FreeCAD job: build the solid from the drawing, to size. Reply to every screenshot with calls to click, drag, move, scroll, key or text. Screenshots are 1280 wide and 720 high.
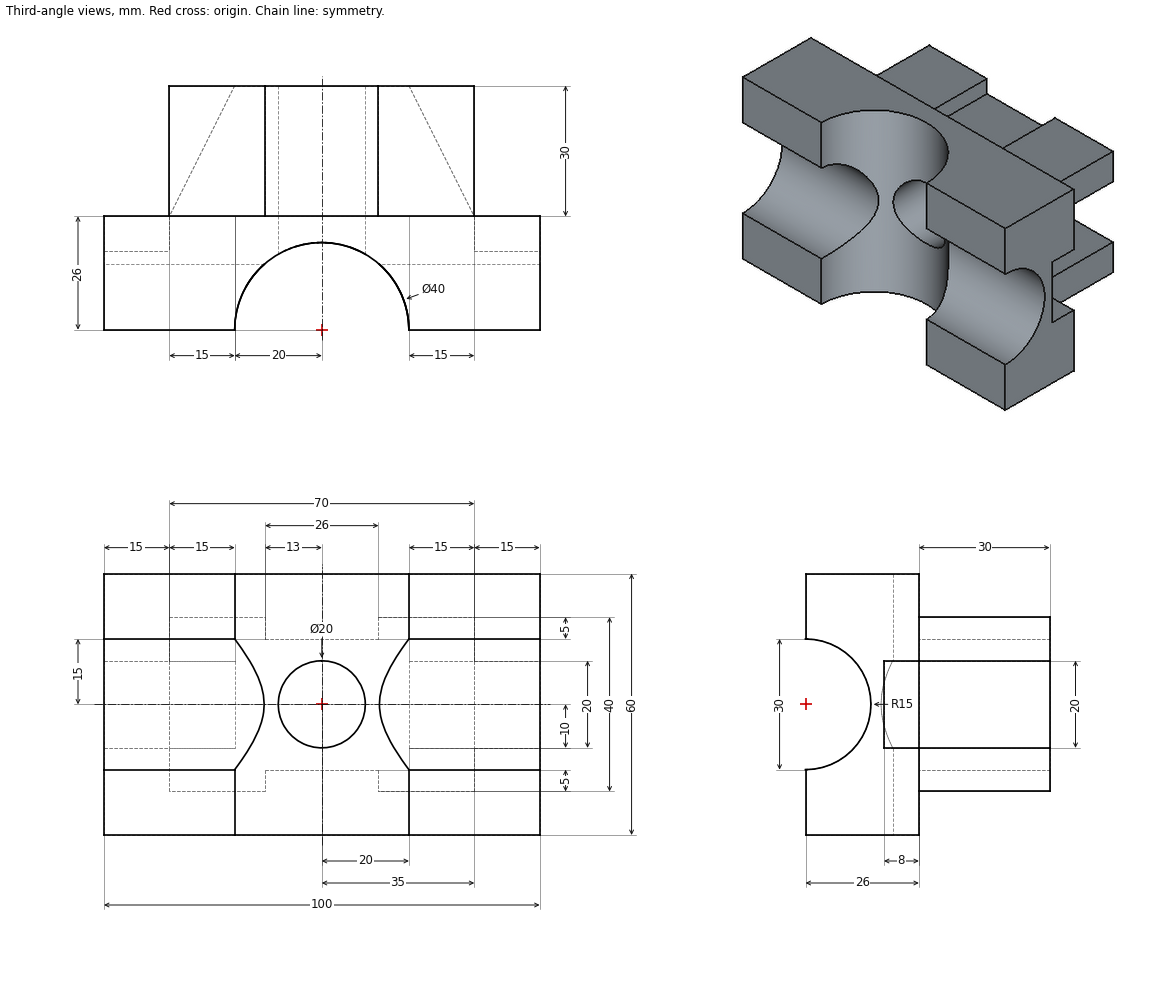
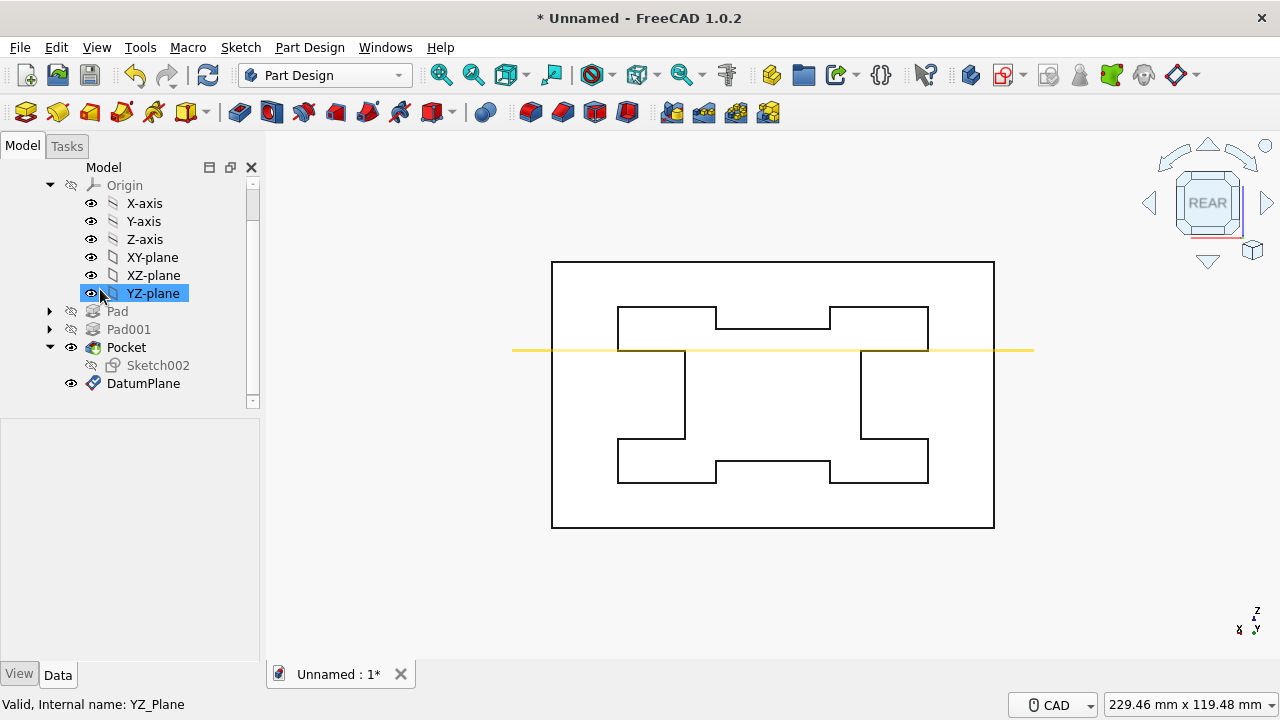
click(116, 383)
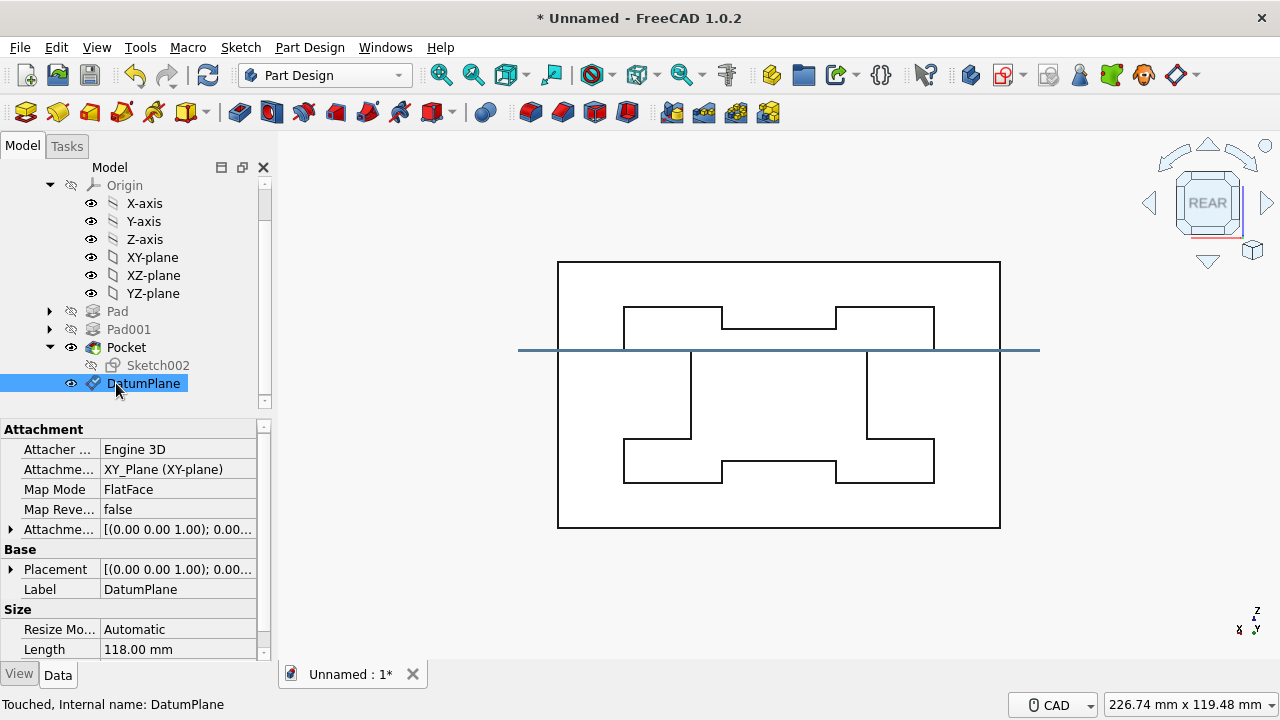
click(1004, 76)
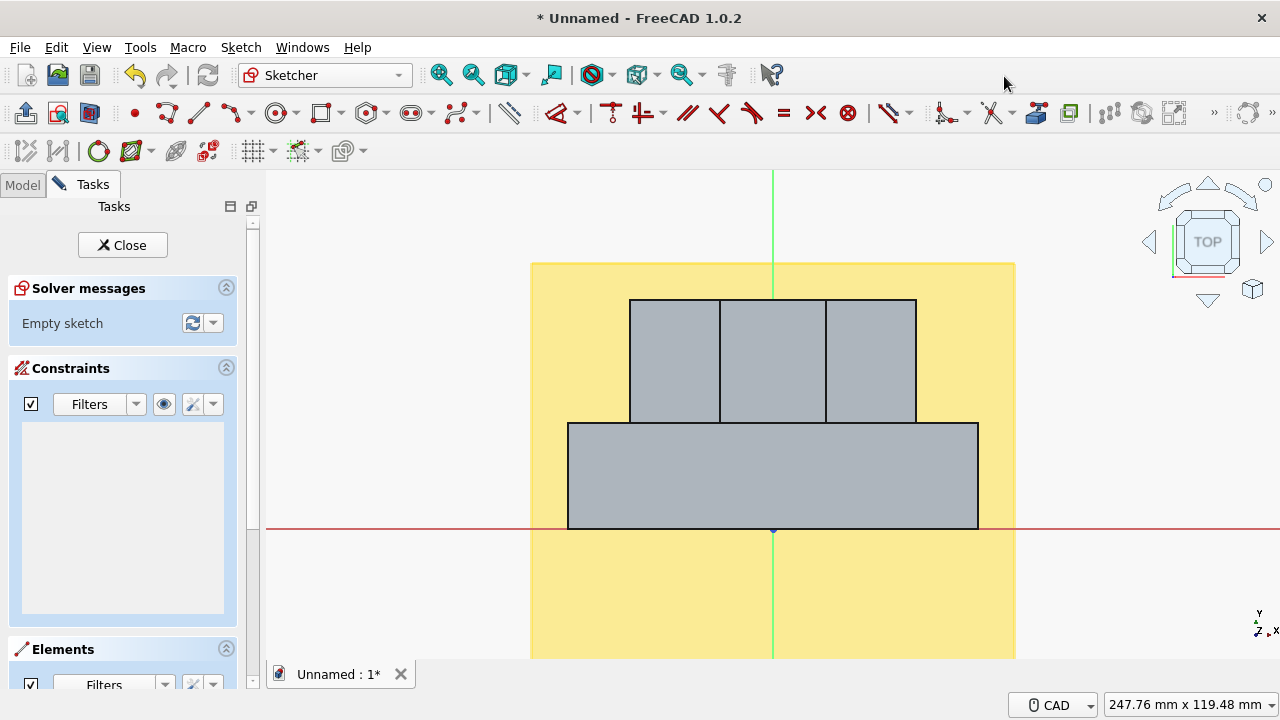
click(90, 114)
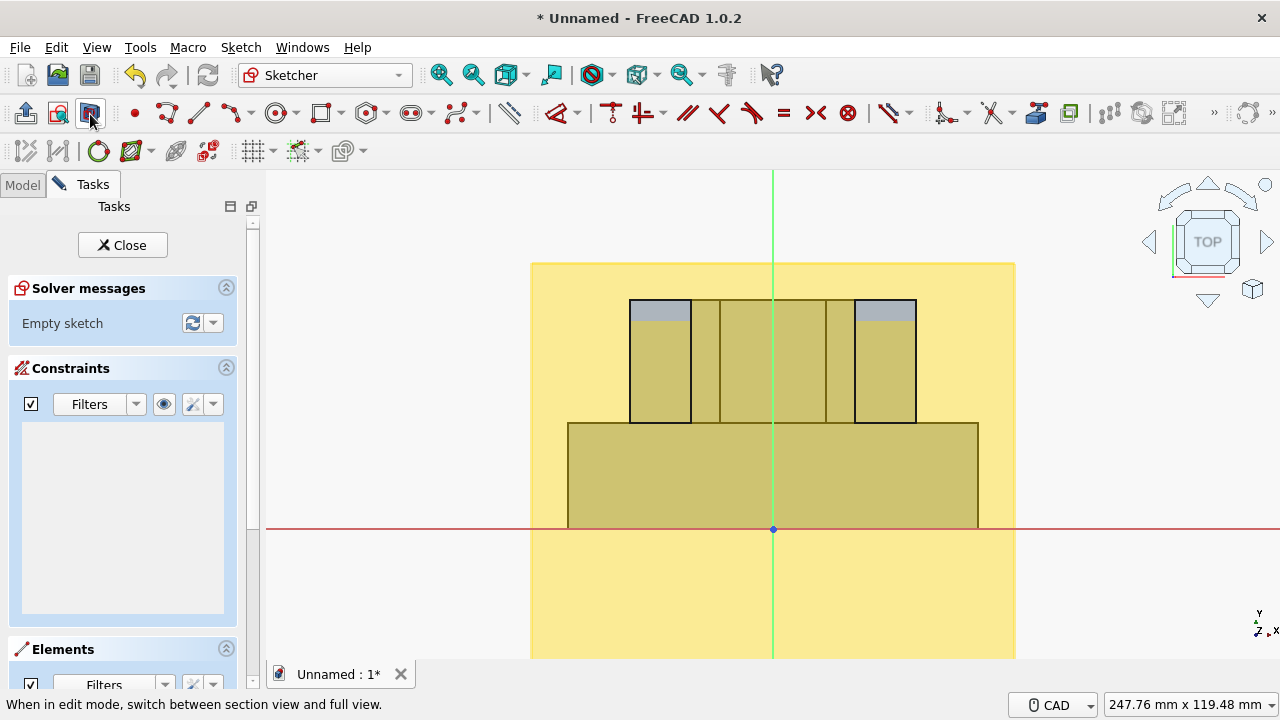
key(g)
key(m)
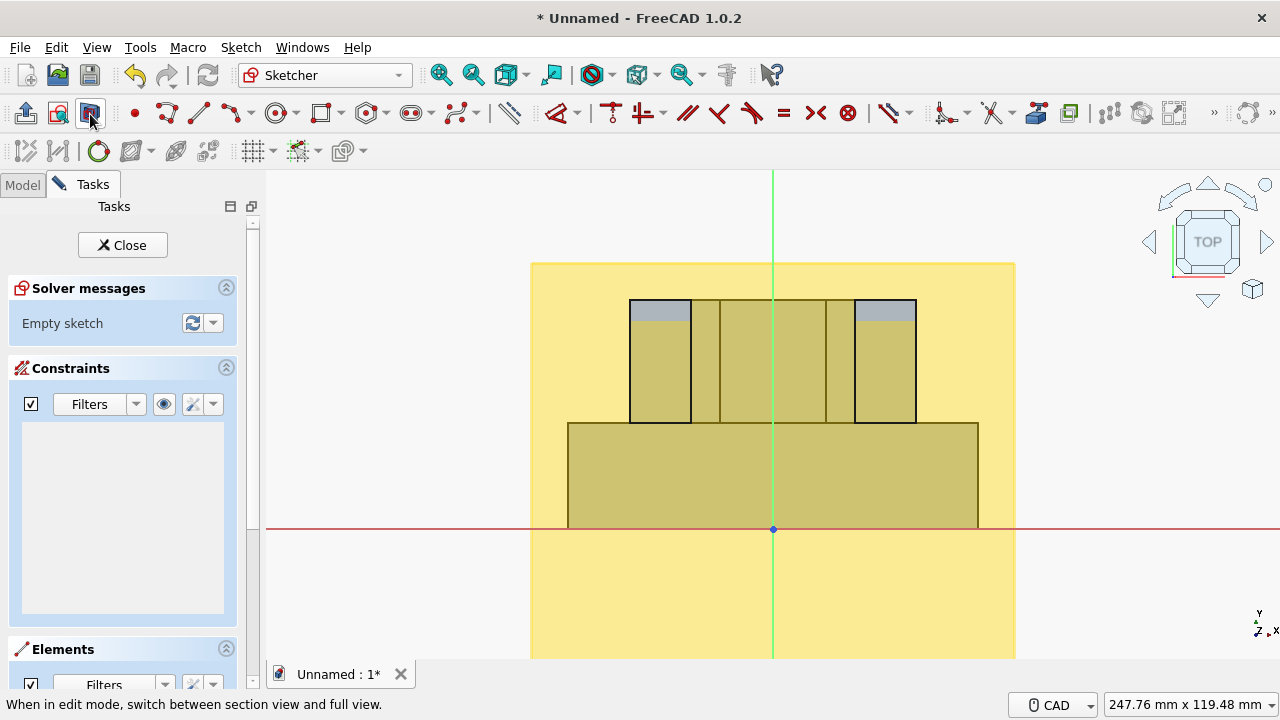
click(691, 423)
click(691, 300)
click(630, 423)
click(691, 424)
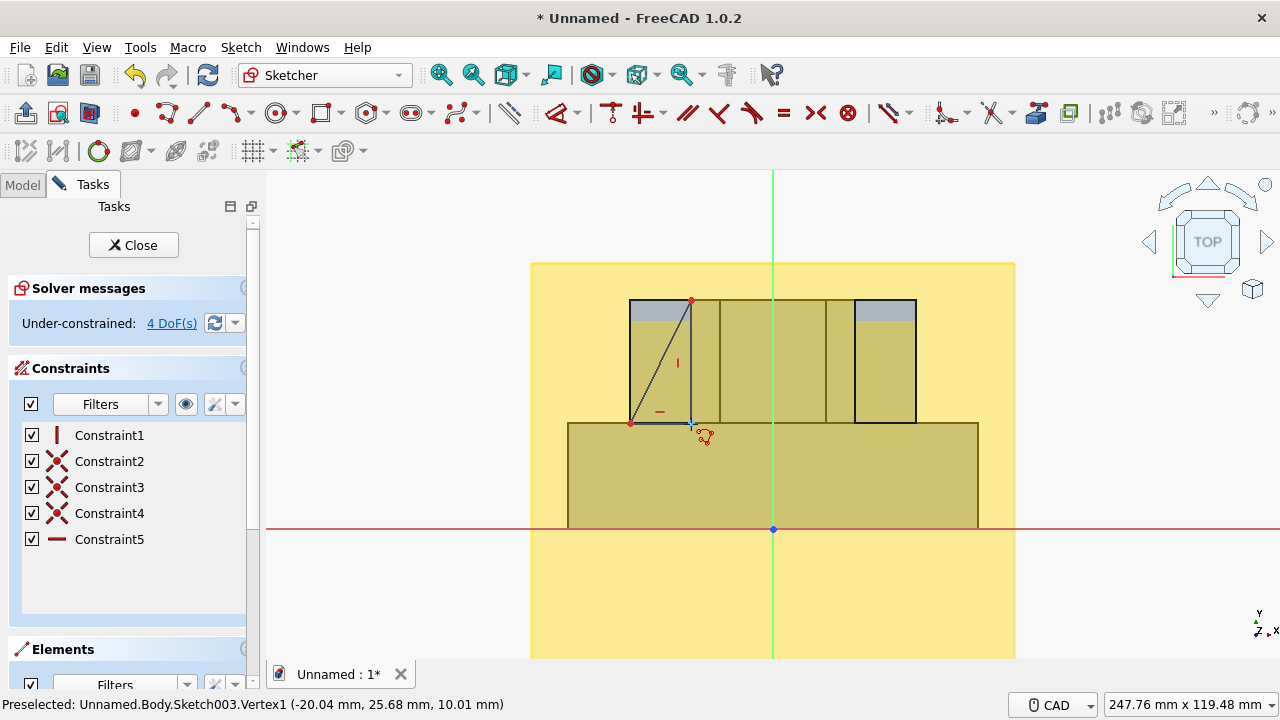
click(855, 423)
click(916, 423)
click(855, 300)
click(855, 424)
key(Escape)
key(Escape)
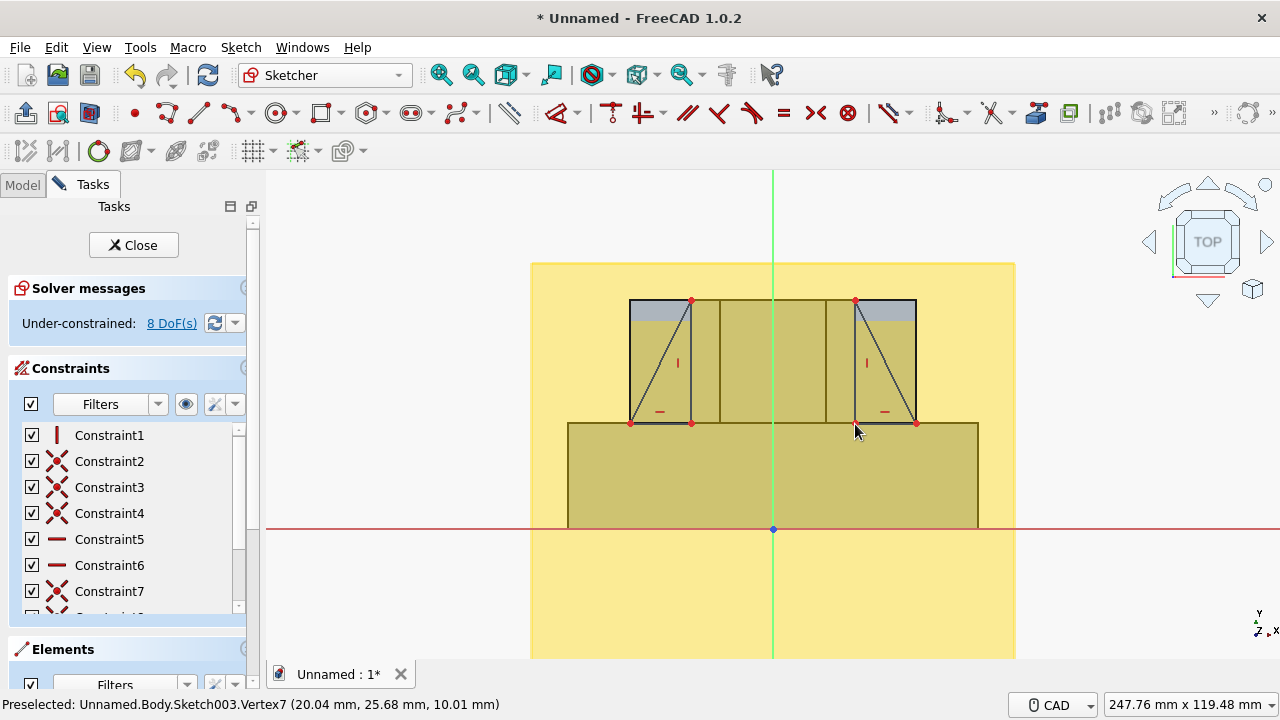
click(691, 424)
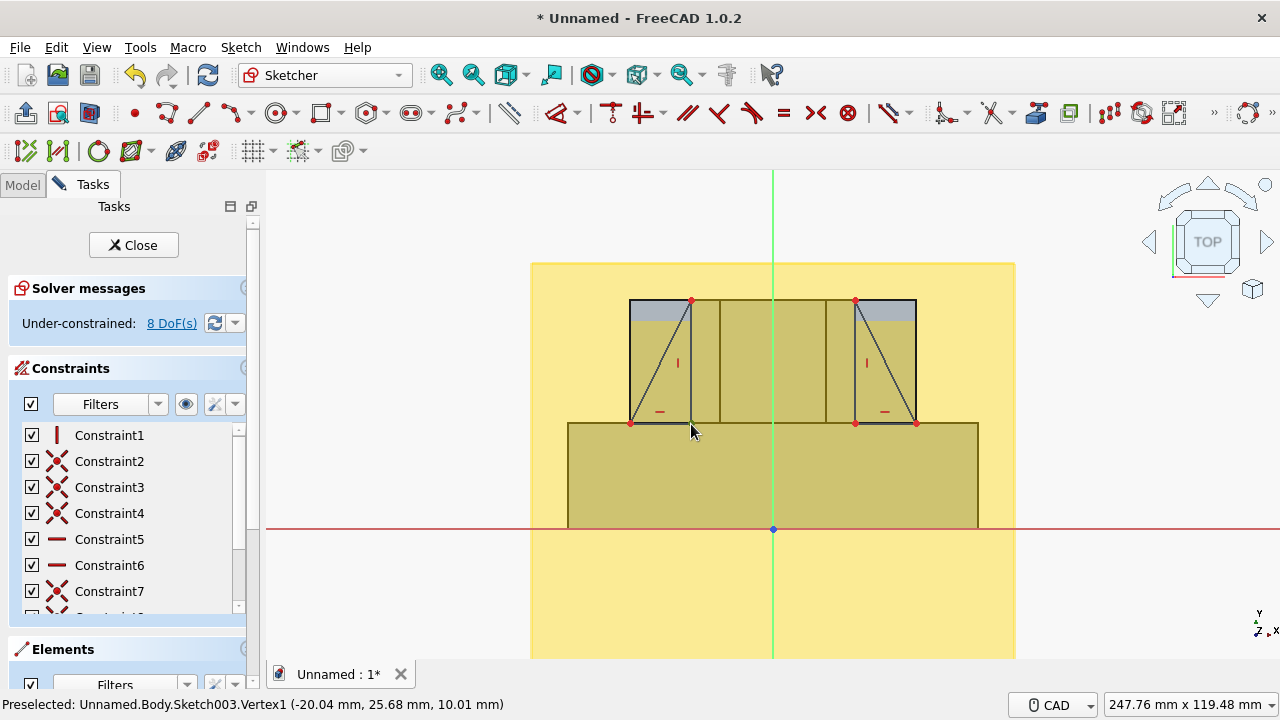
click(855, 424)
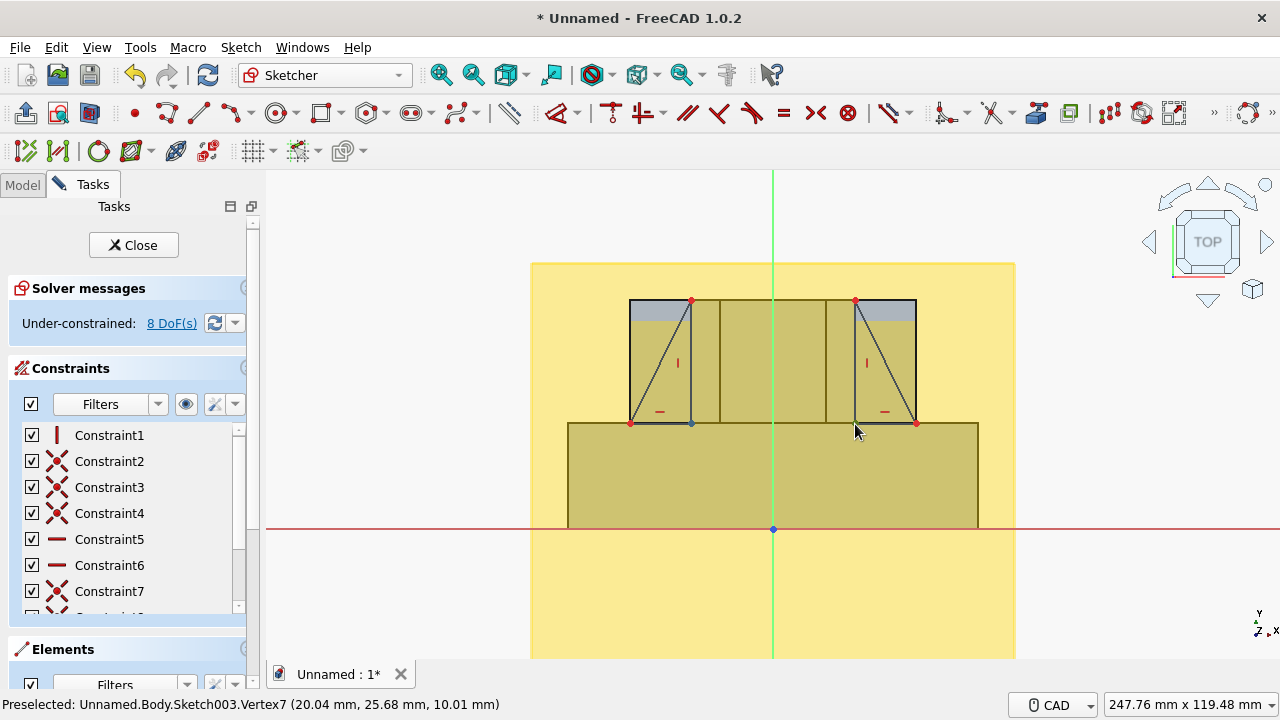
click(773, 600)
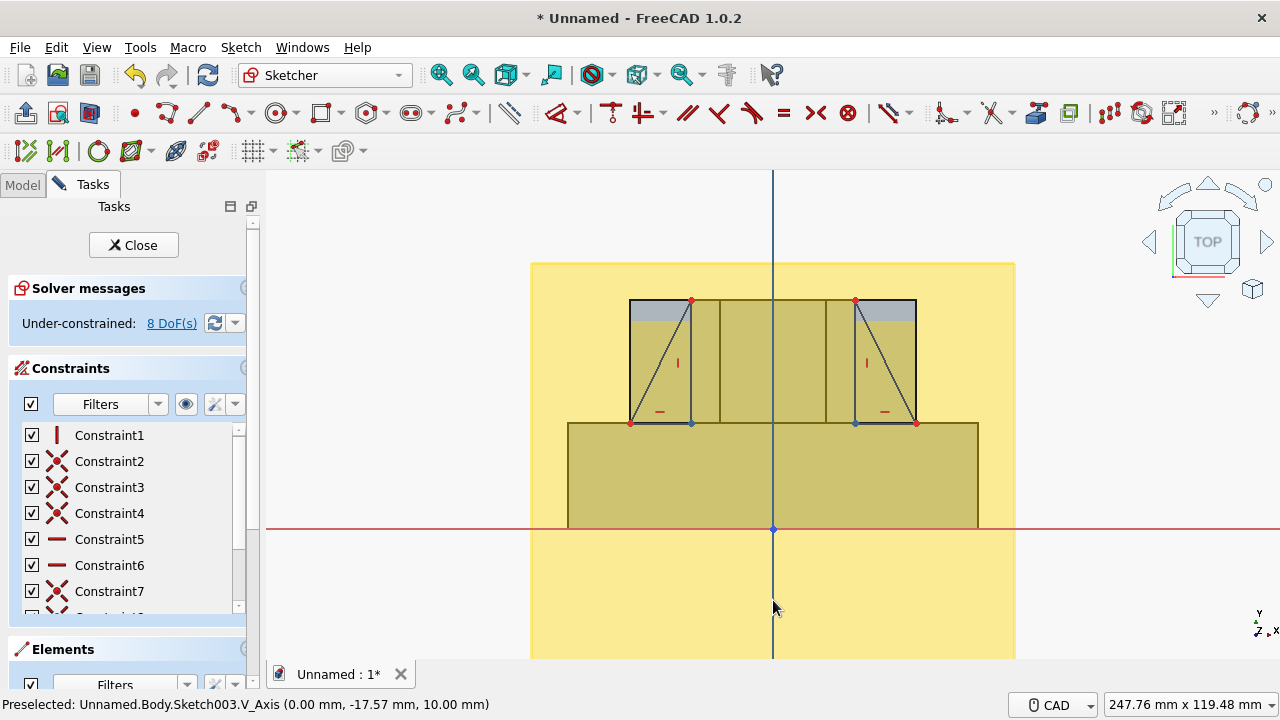
click(816, 114)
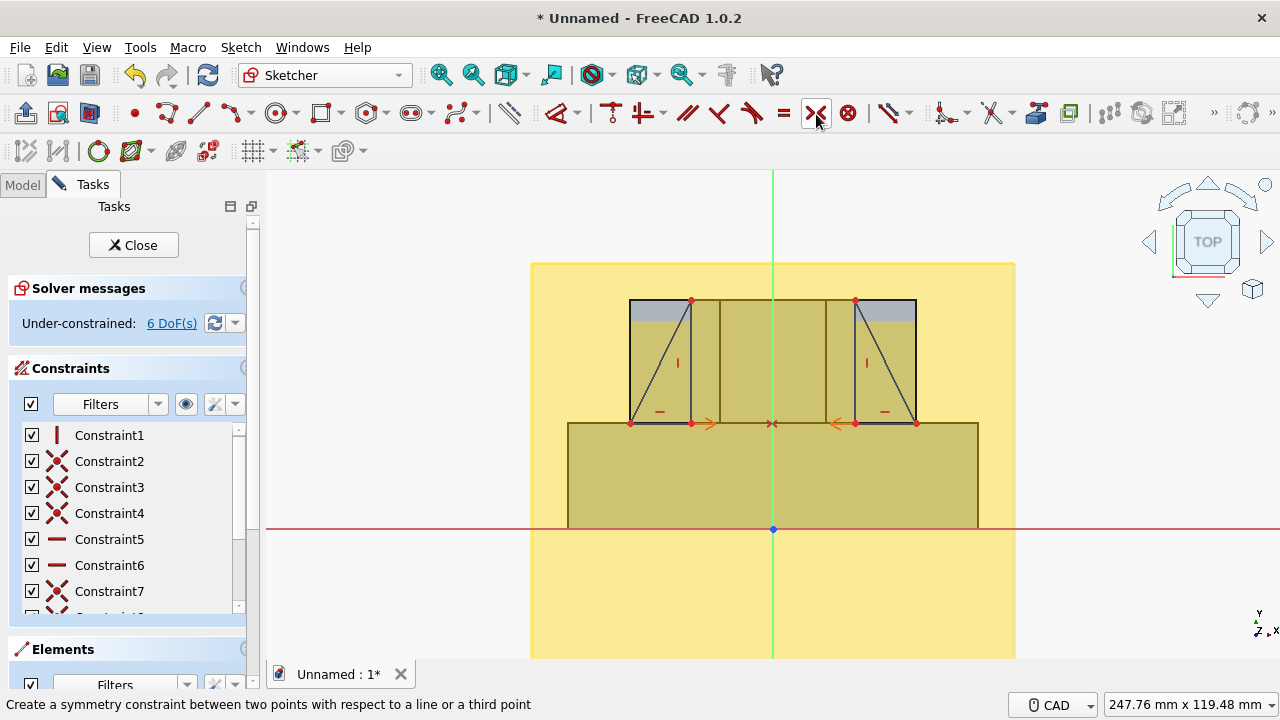
key(d)